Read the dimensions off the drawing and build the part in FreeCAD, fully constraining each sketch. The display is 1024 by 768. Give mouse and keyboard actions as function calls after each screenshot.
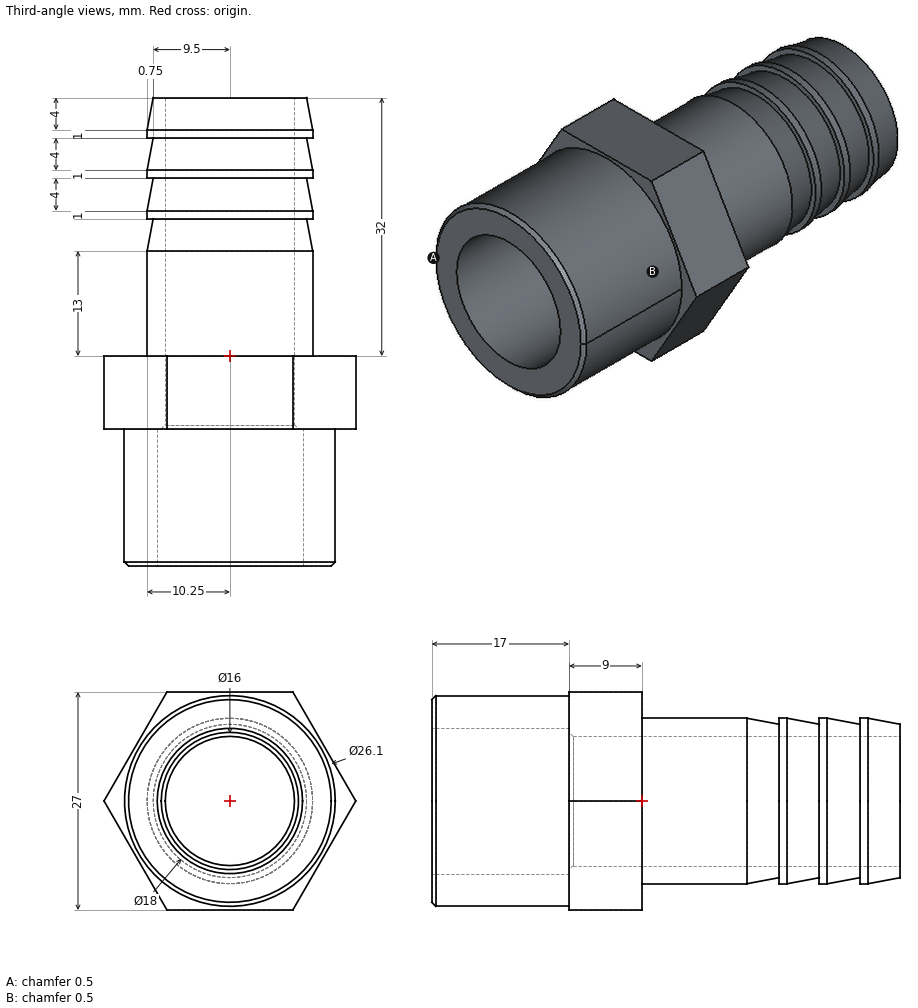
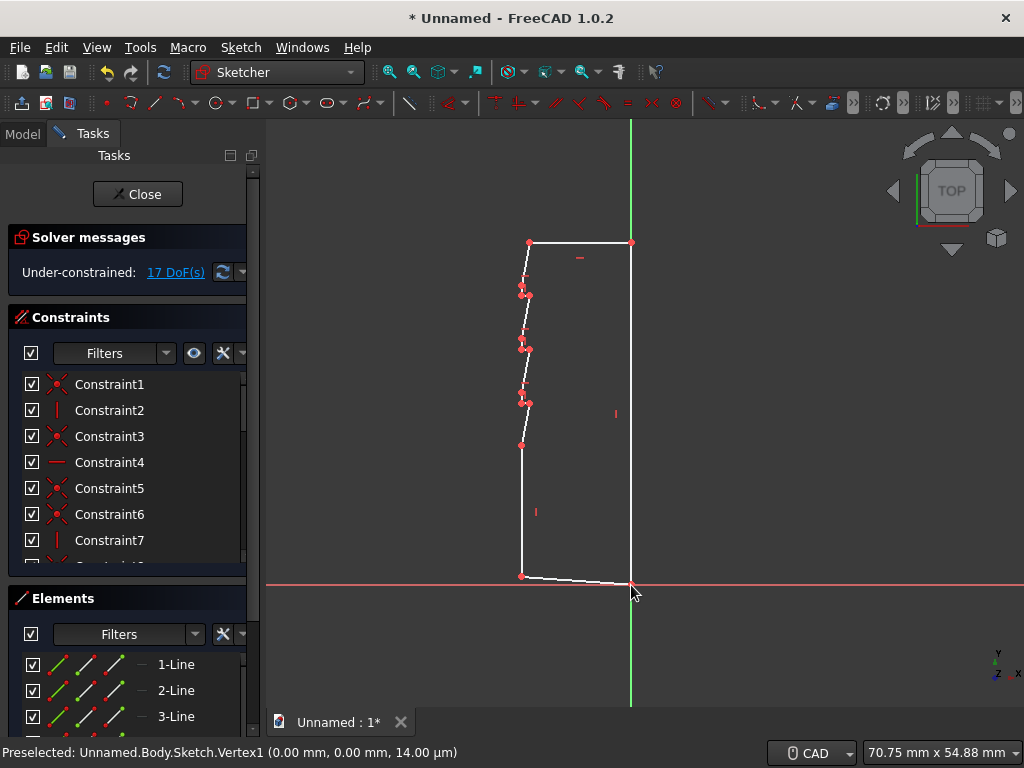
click(599, 582)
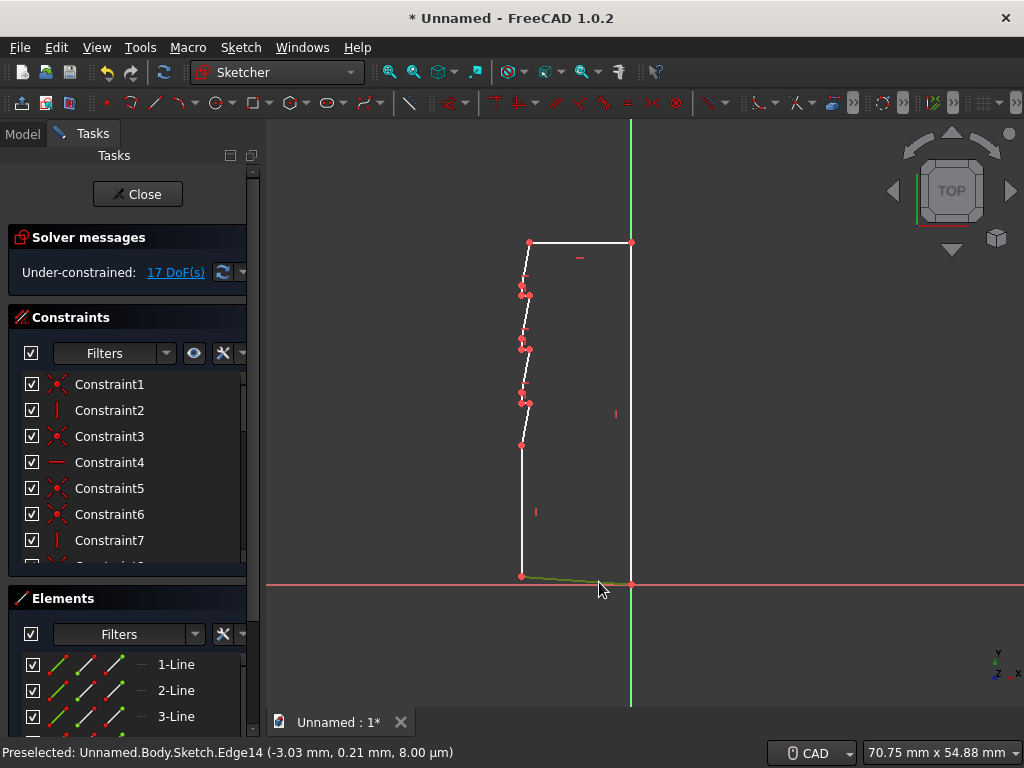
key(h)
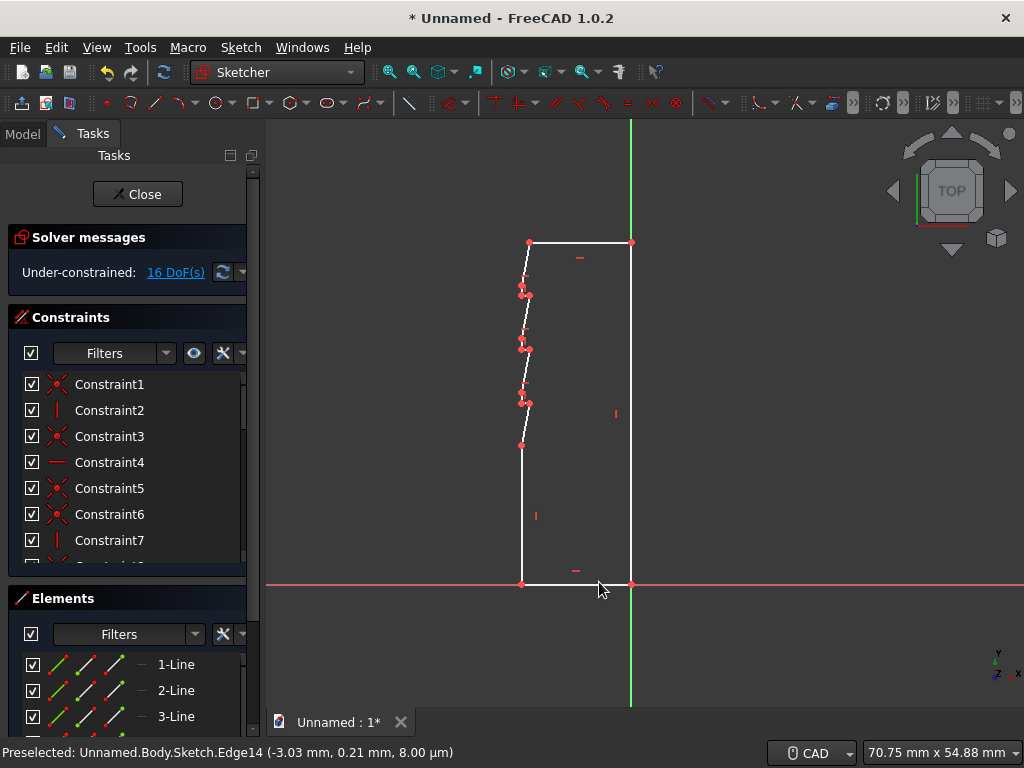
key(d)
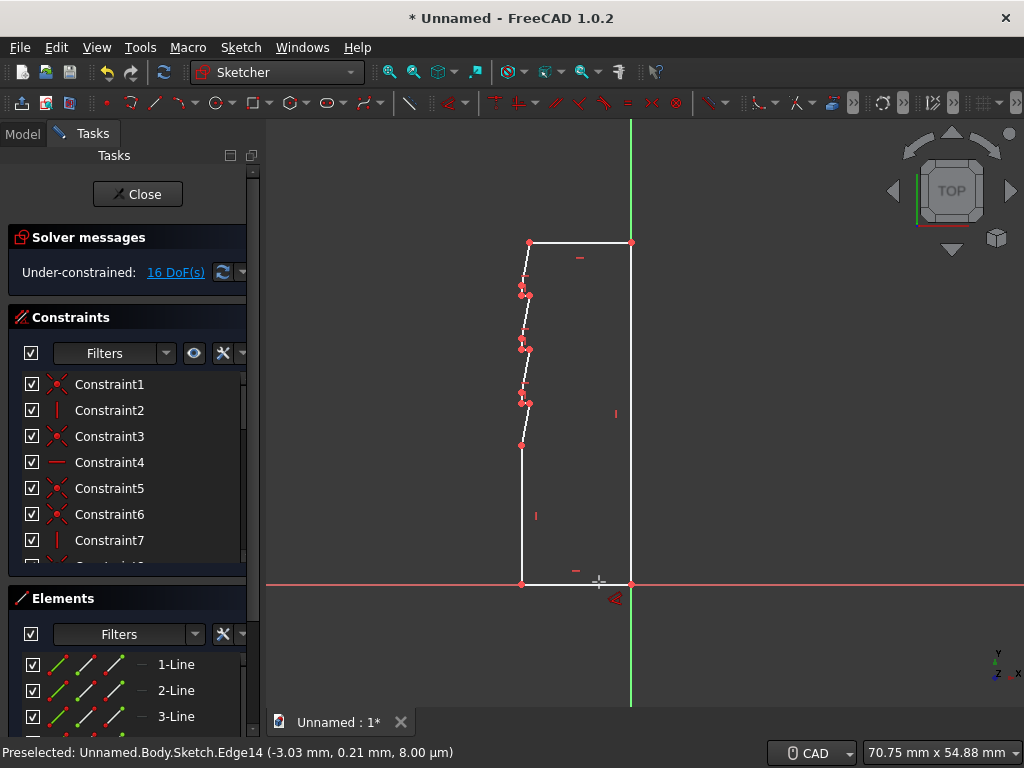
scroll(522, 291, up, 7)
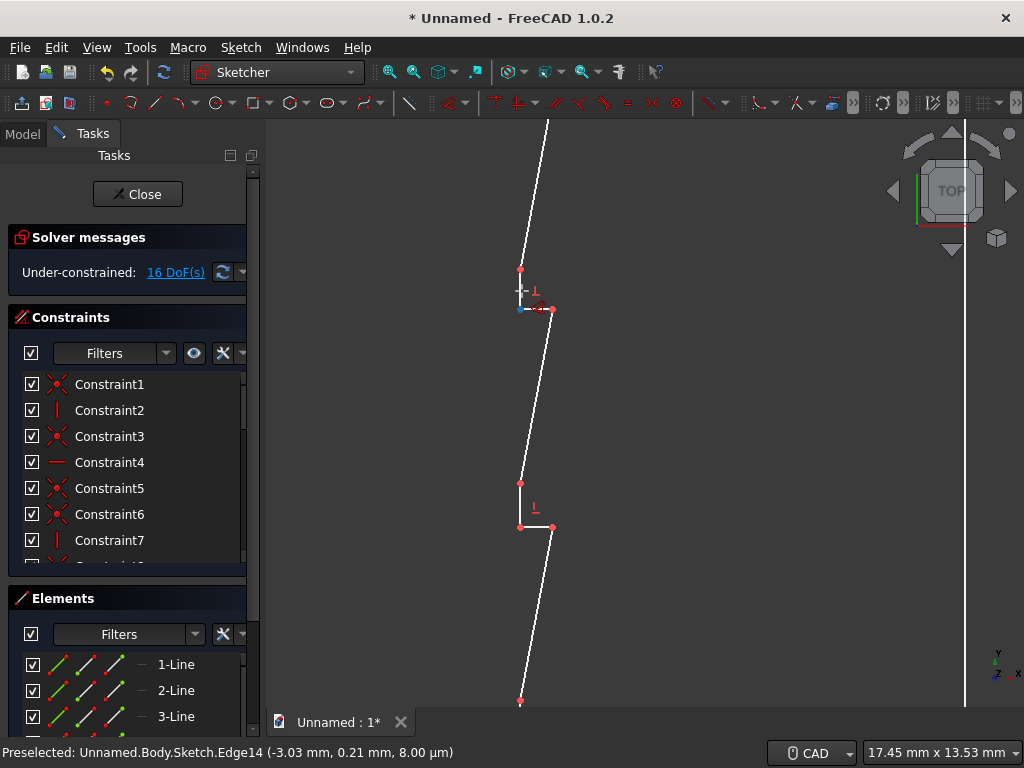
click(520, 290)
click(486, 290)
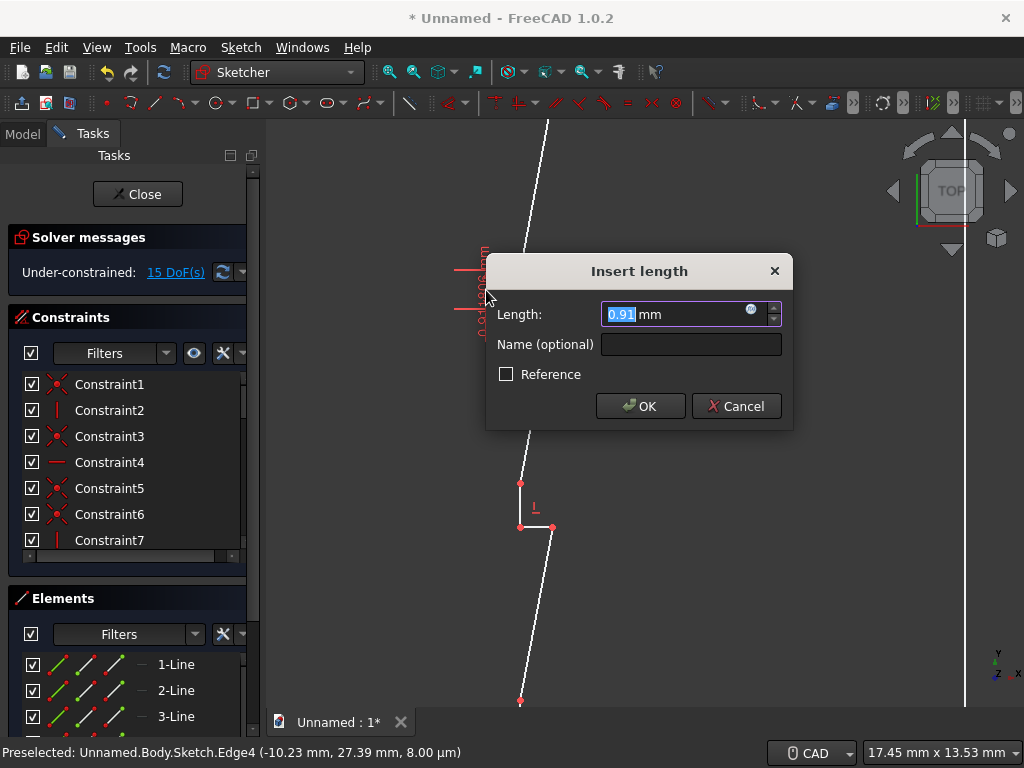
text(1)
key(Return)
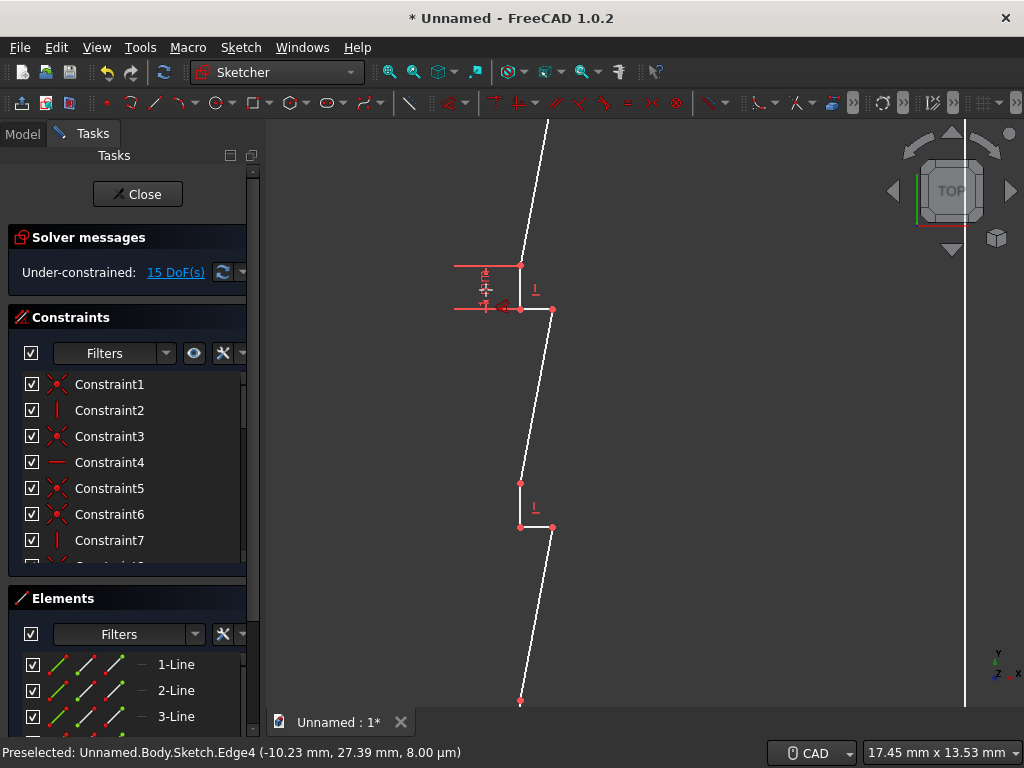
click(520, 497)
click(486, 506)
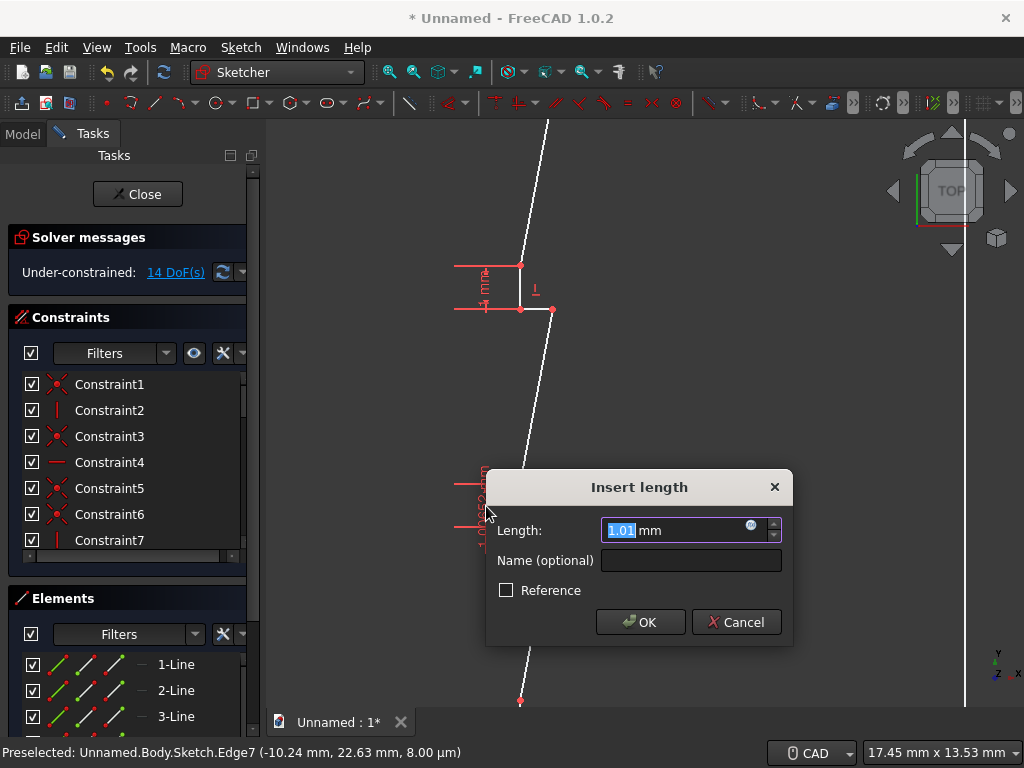
text(1)
key(Return)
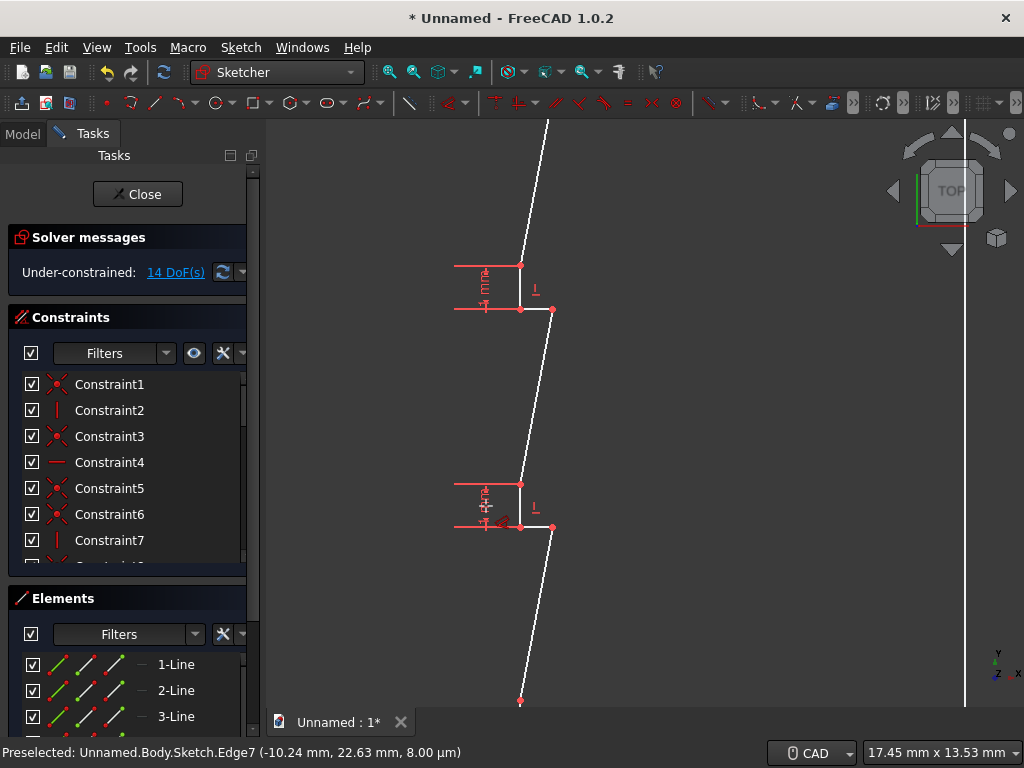
scroll(522, 291, down, 7)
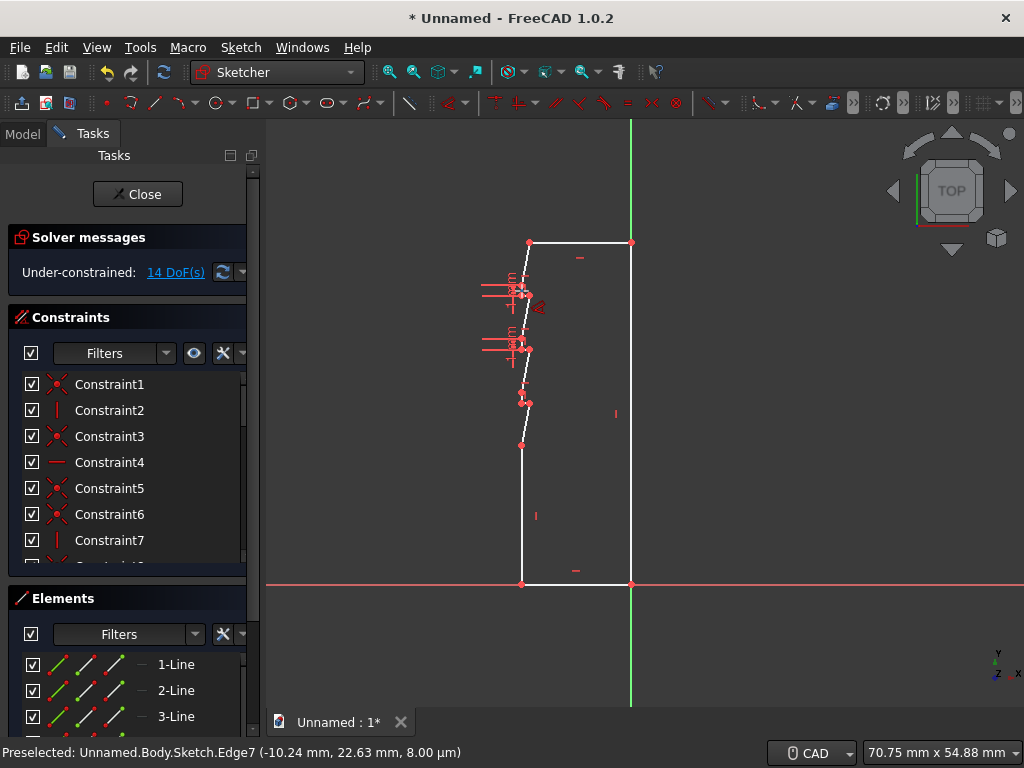
scroll(522, 395, up, 8)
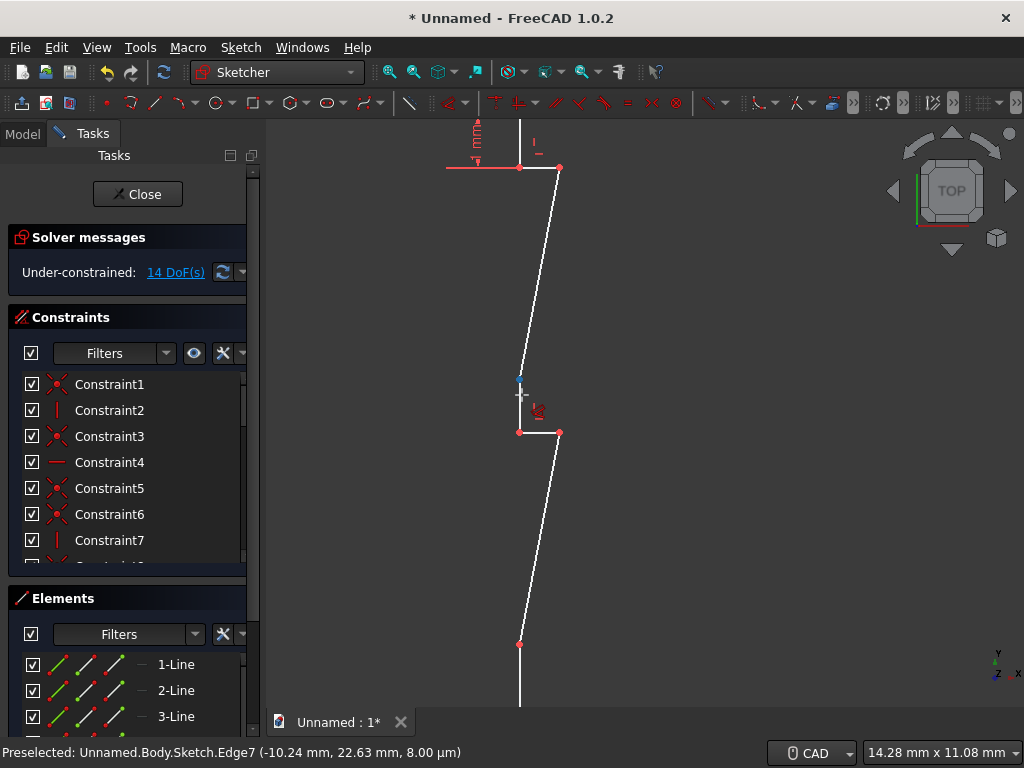
click(520, 395)
click(486, 406)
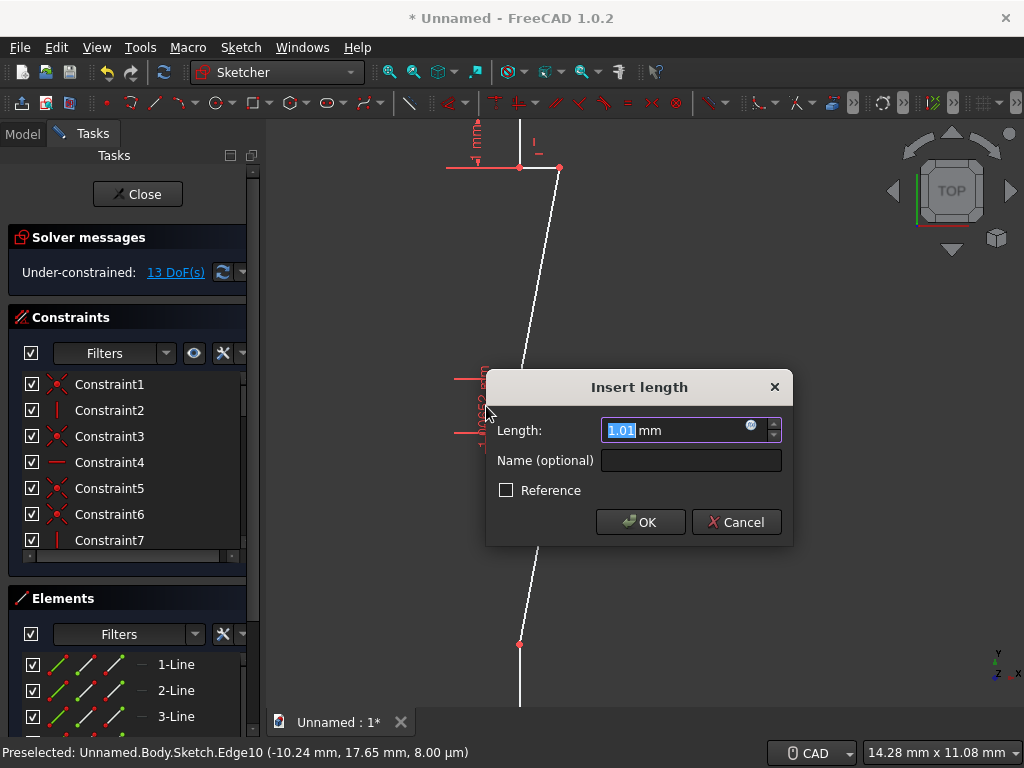
text(1)
key(Return)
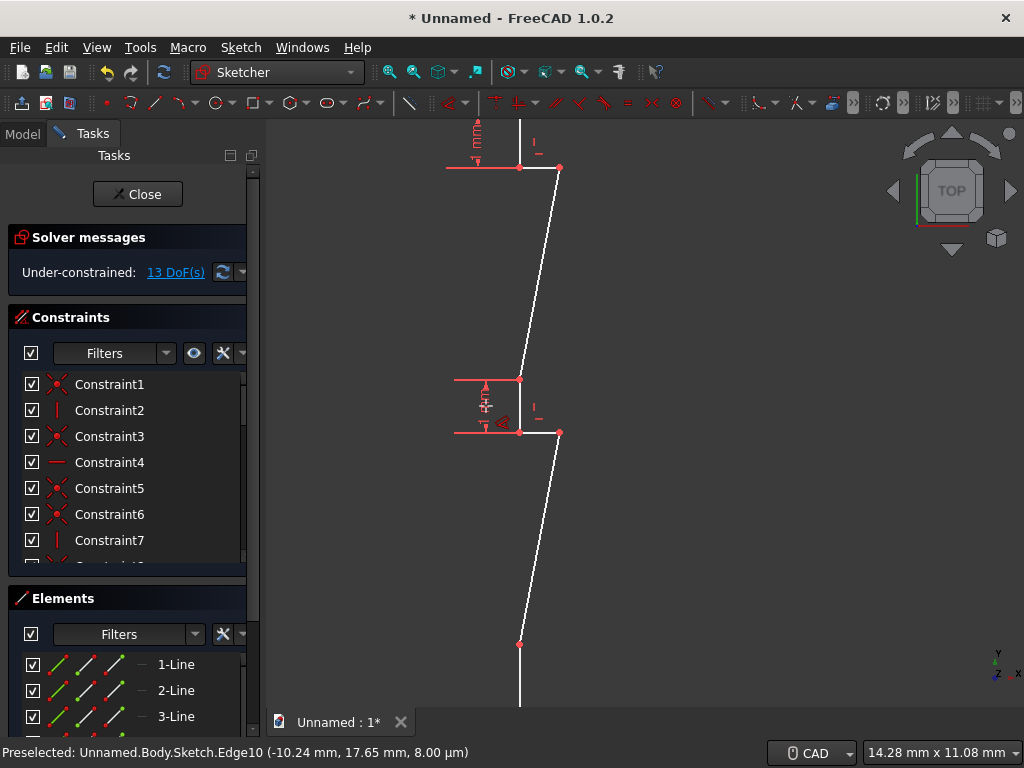
scroll(522, 395, down, 8)